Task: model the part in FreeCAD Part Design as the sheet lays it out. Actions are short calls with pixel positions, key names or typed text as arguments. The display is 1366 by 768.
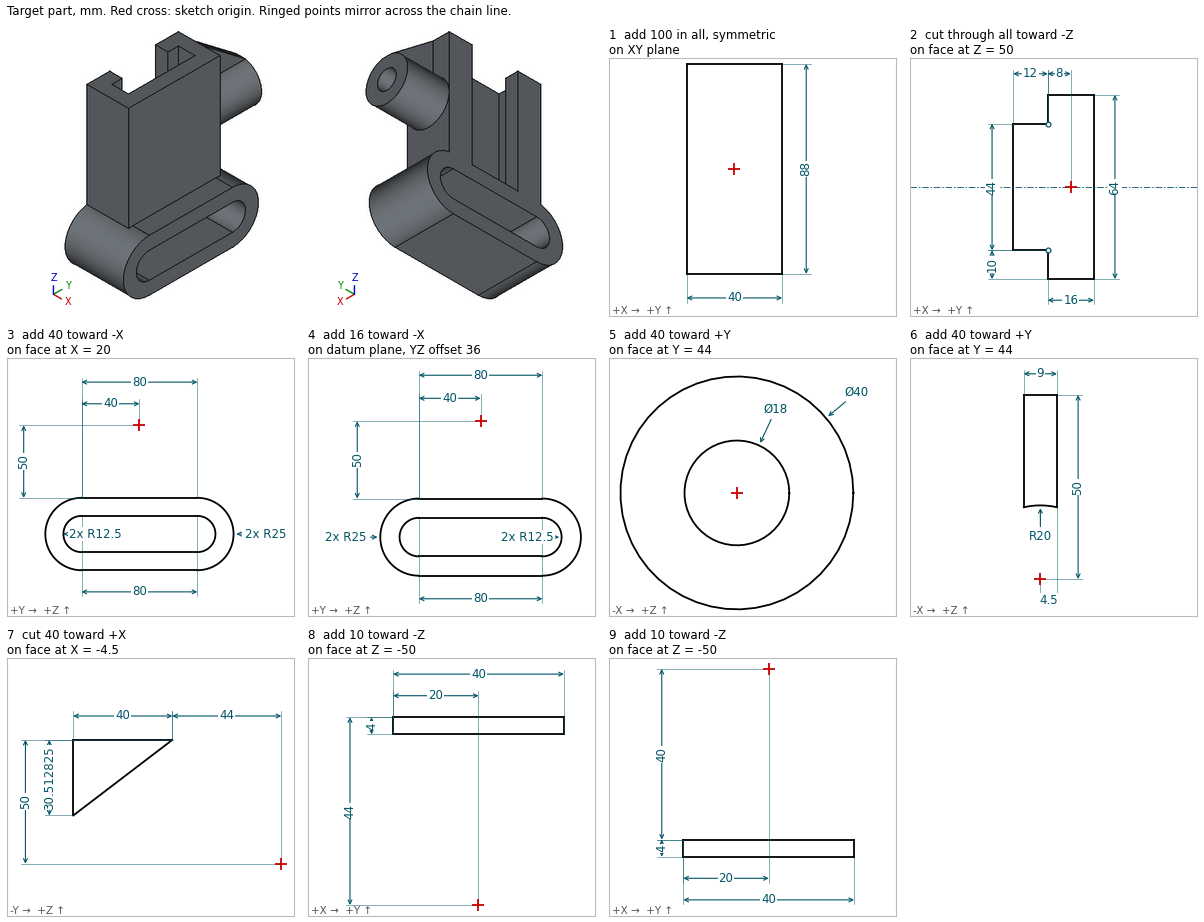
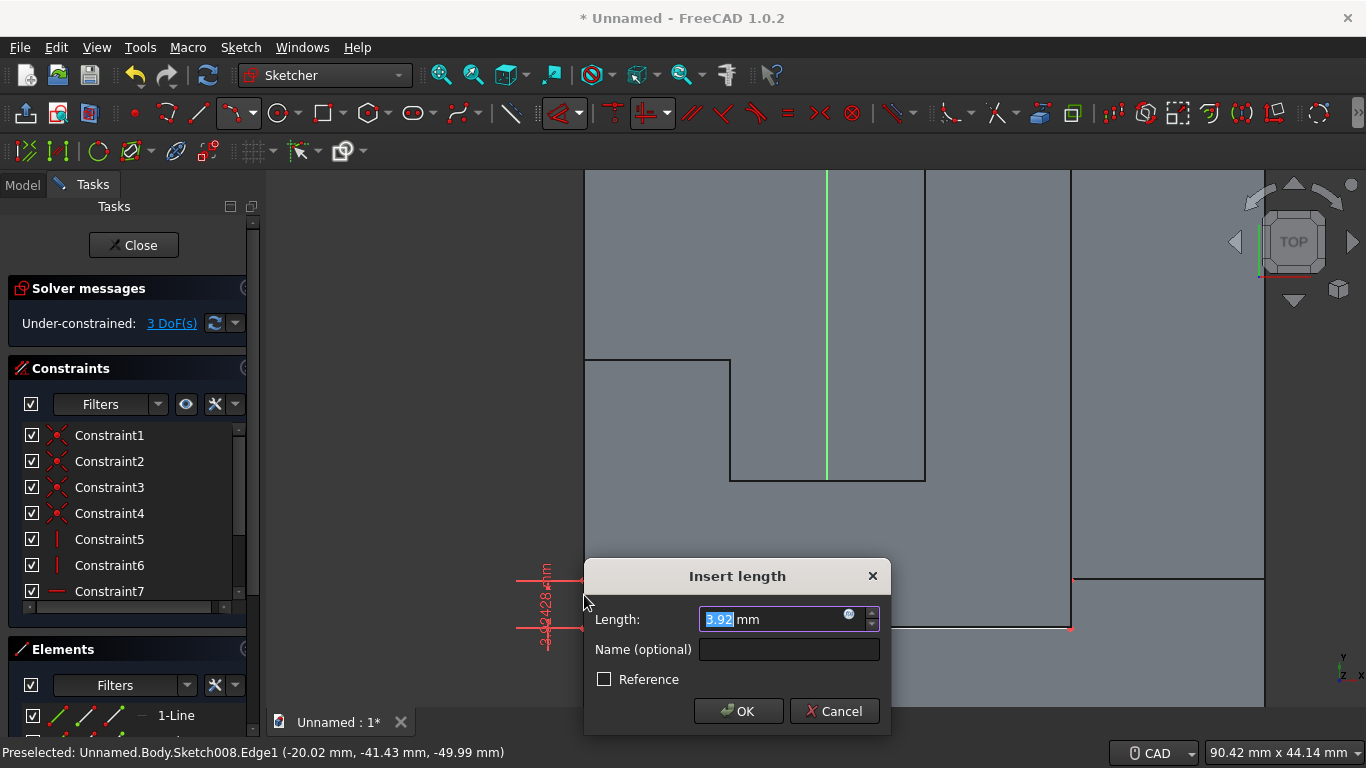
text(4)
key(Return)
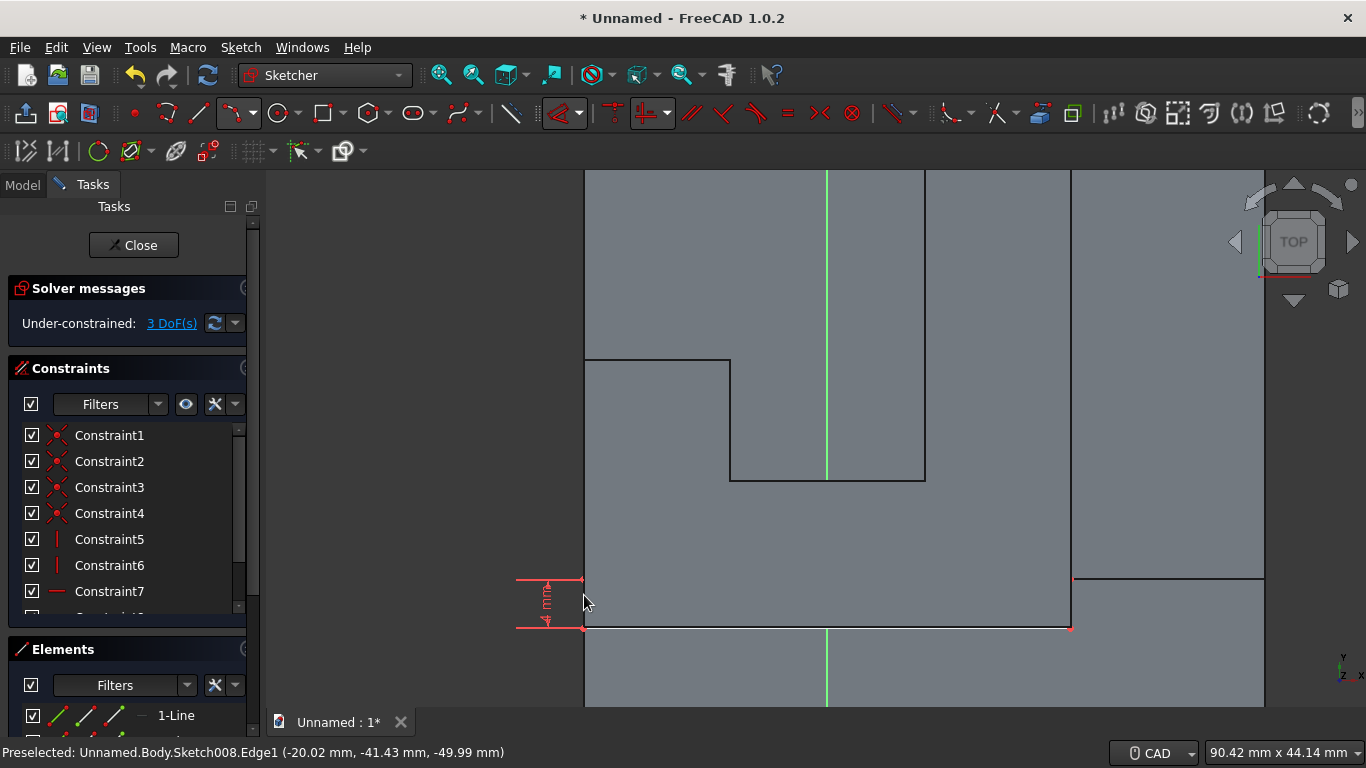
click(730, 628)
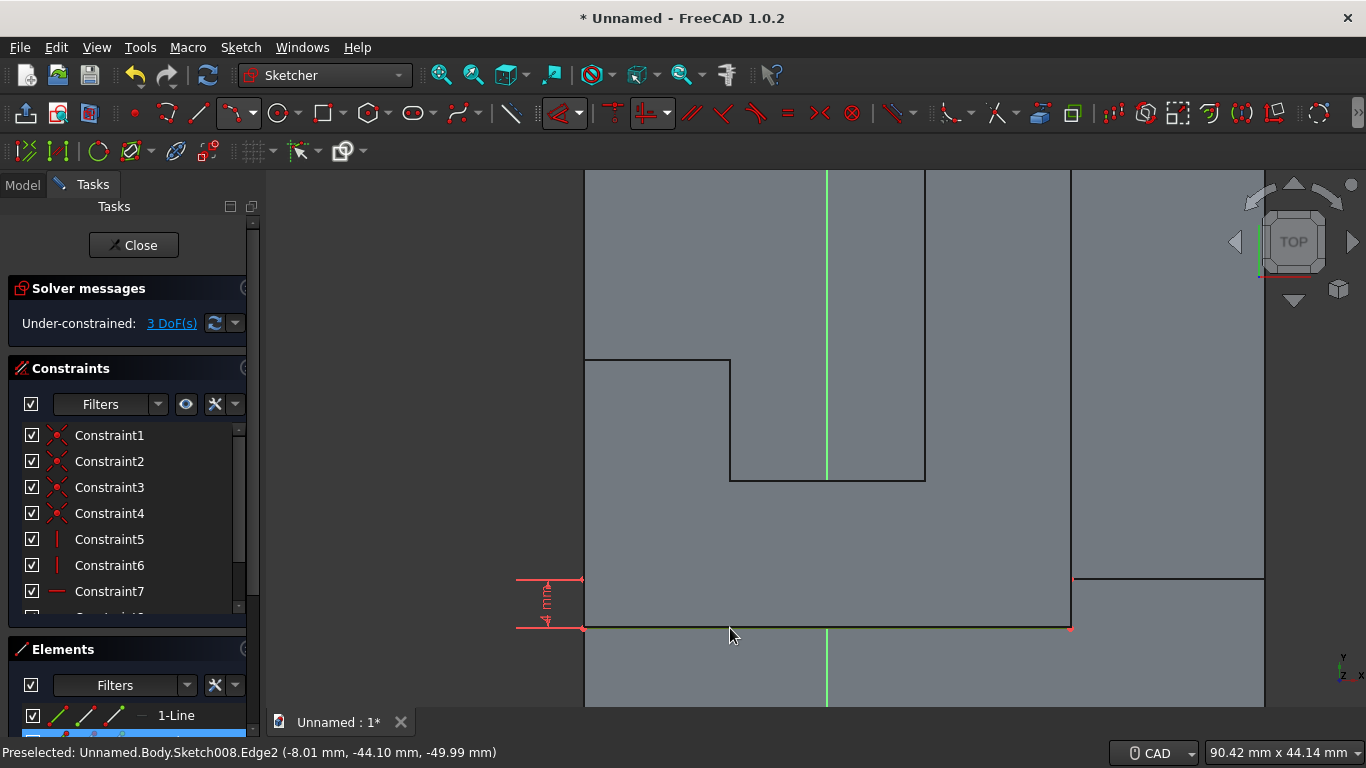
key(l)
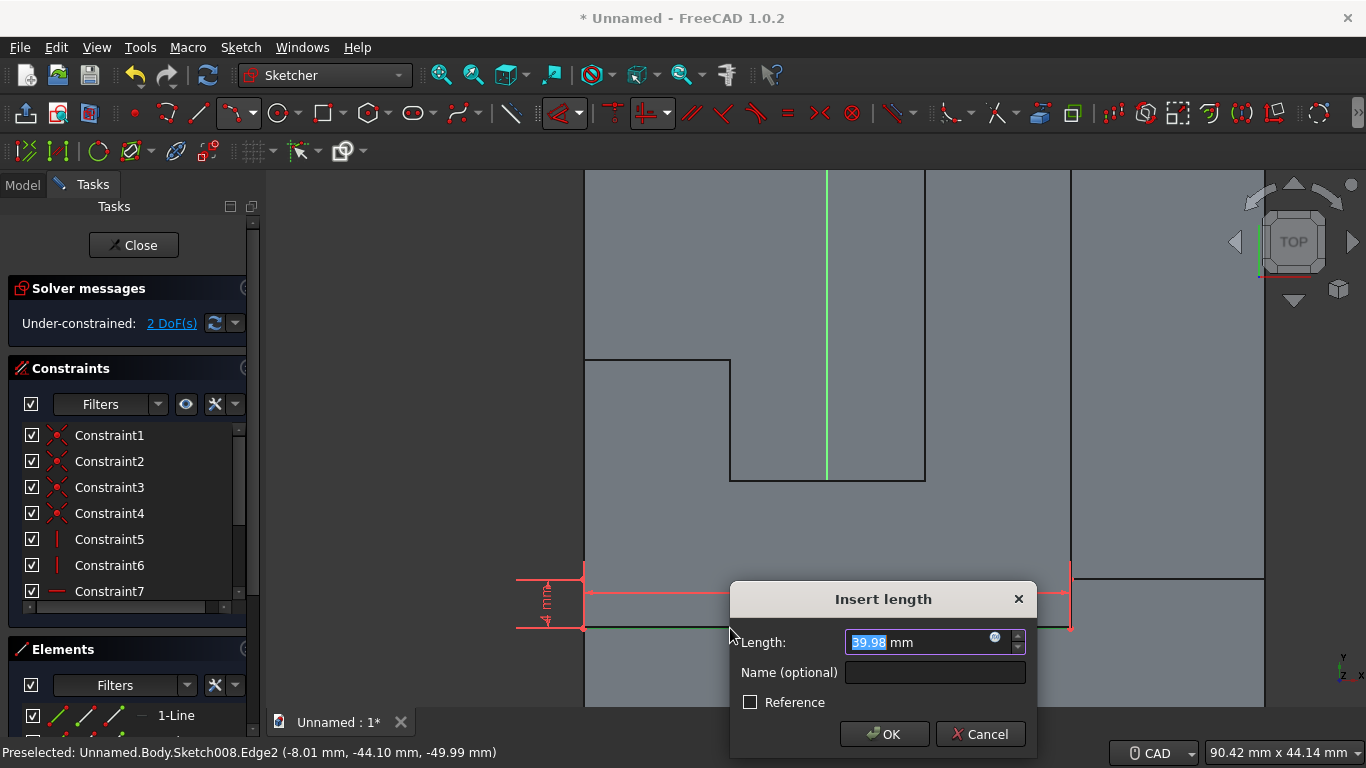
text(40)
key(Return)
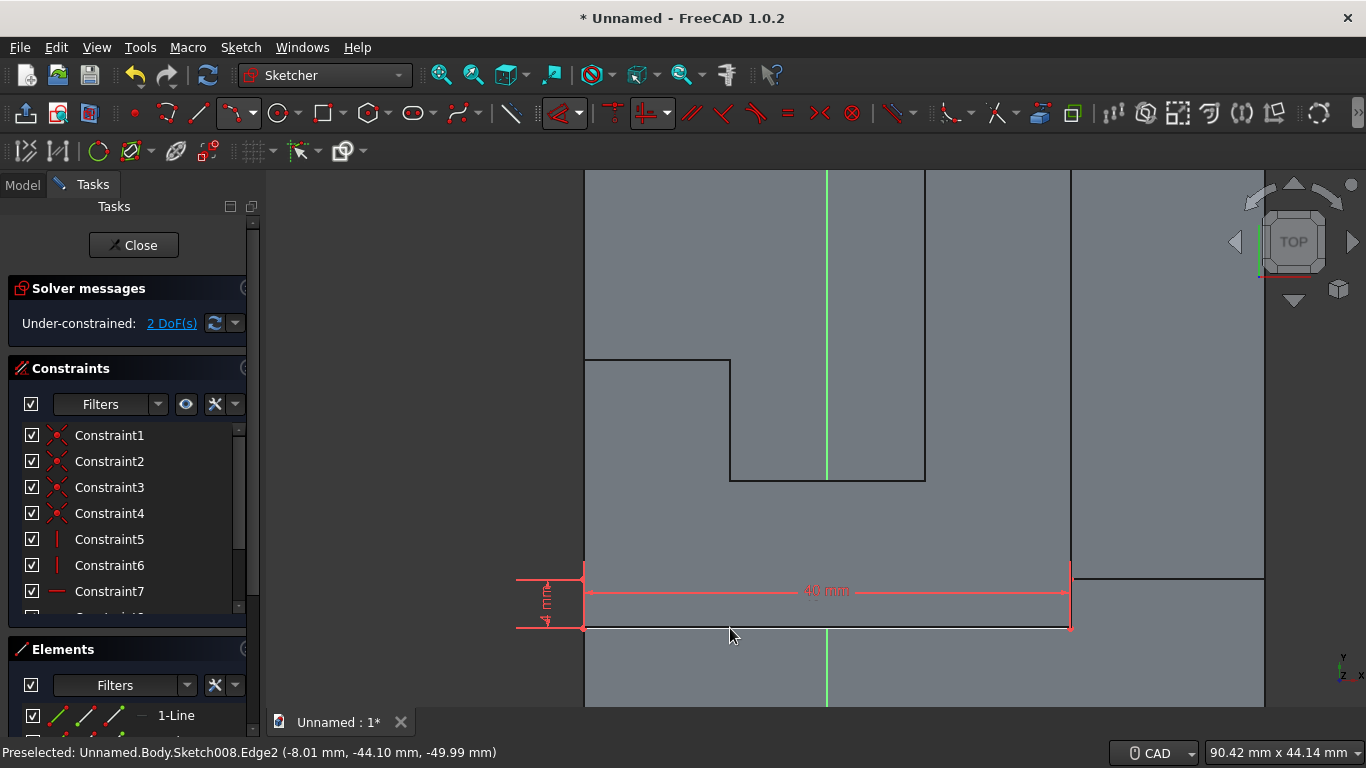
click(584, 580)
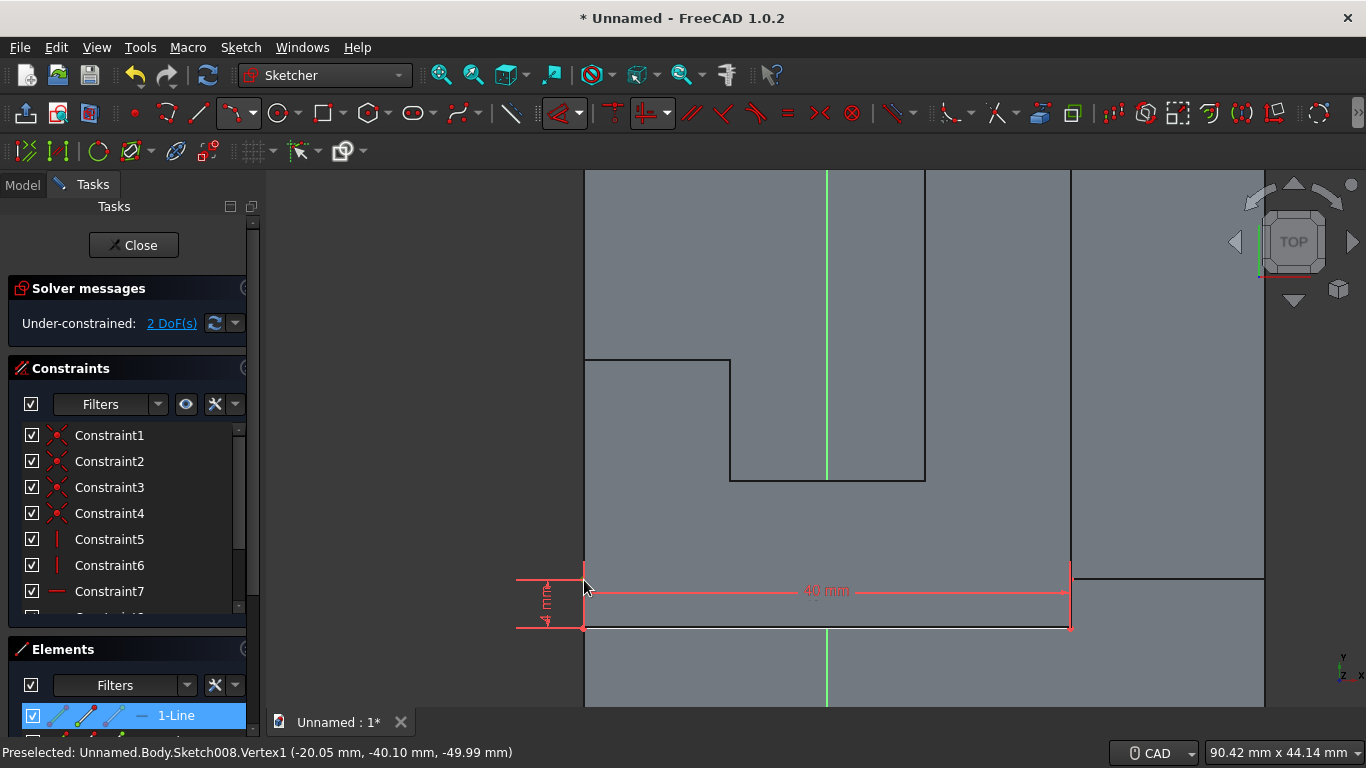
key(l)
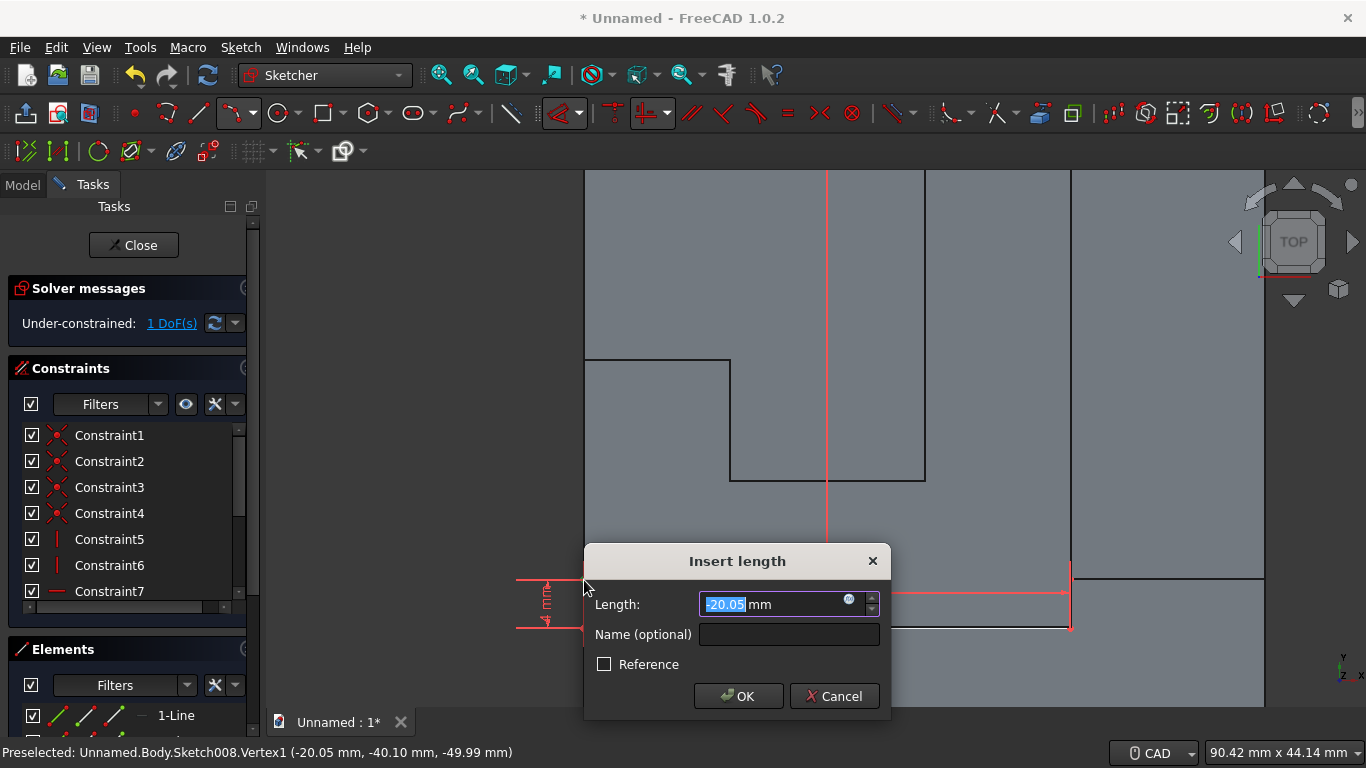
text(-20)
key(Return)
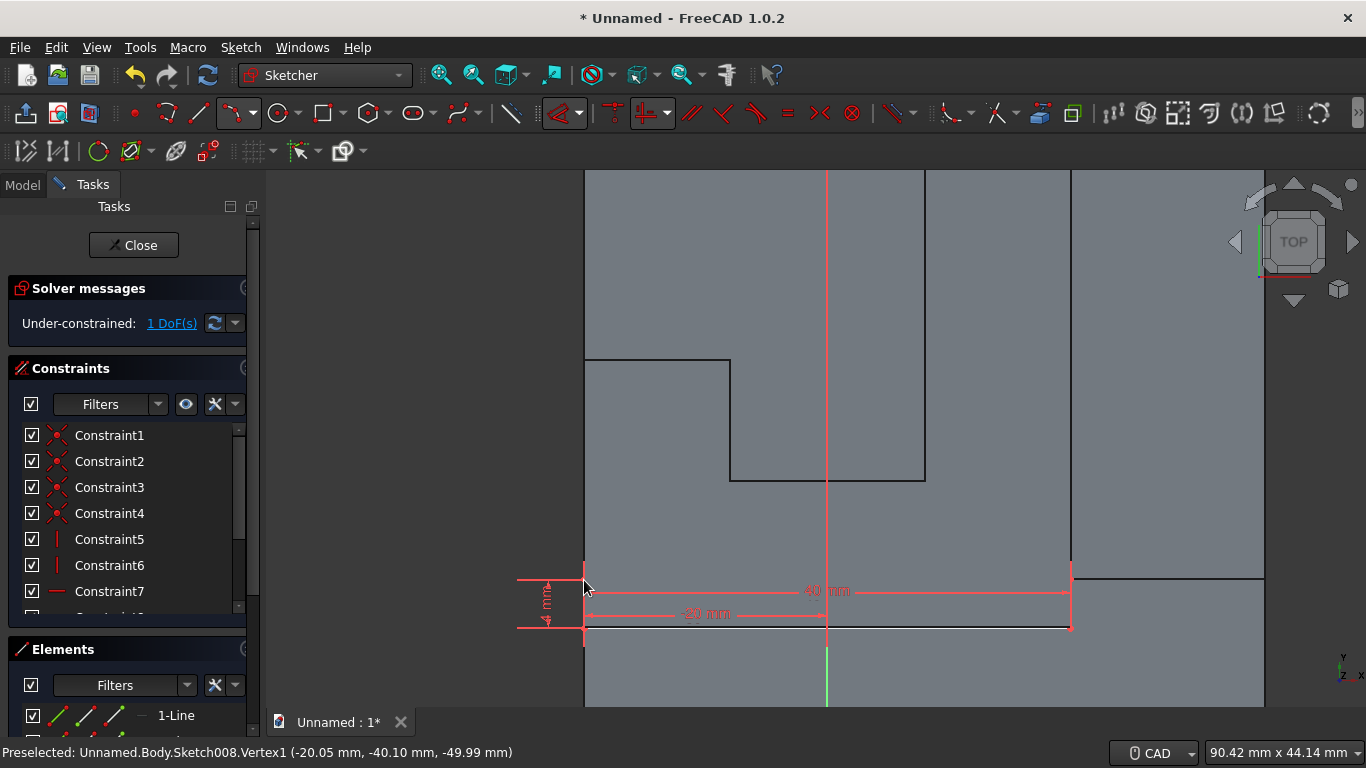
click(584, 580)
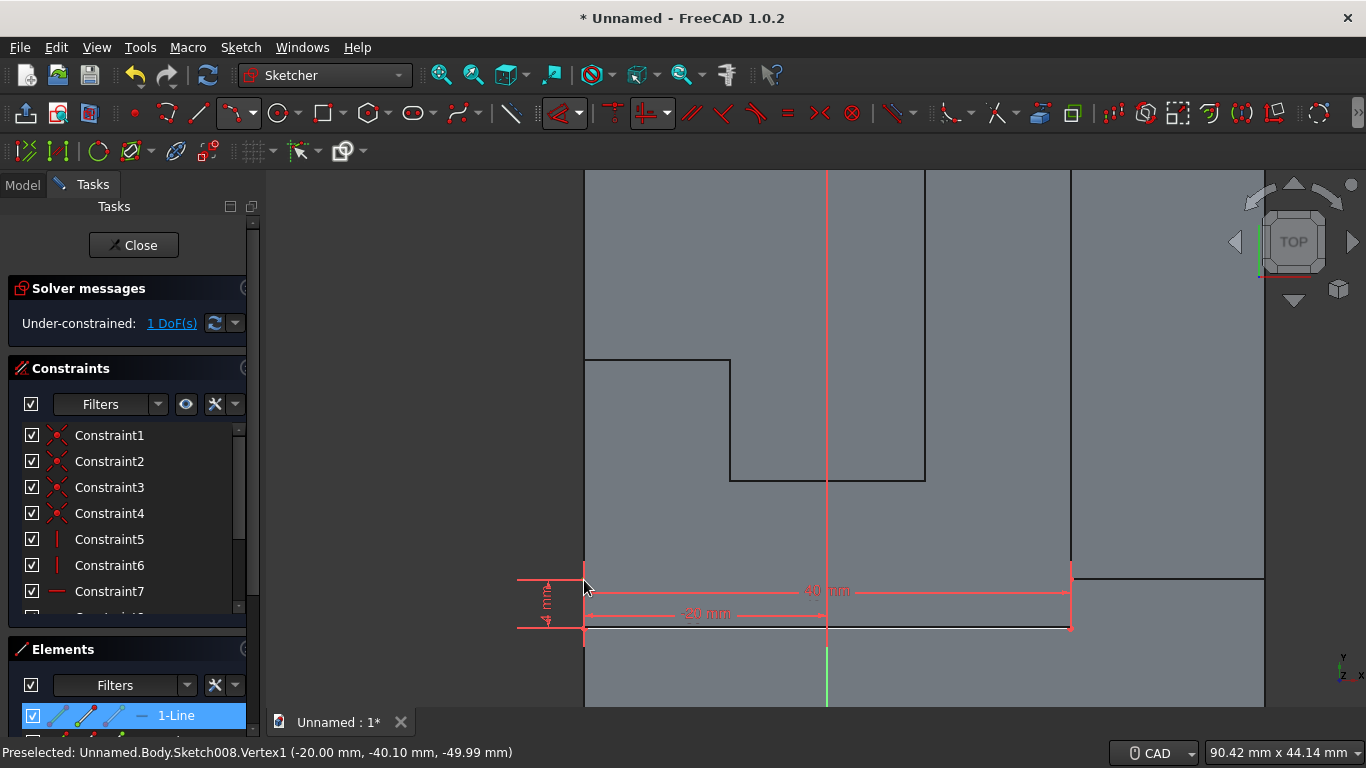
key(i)